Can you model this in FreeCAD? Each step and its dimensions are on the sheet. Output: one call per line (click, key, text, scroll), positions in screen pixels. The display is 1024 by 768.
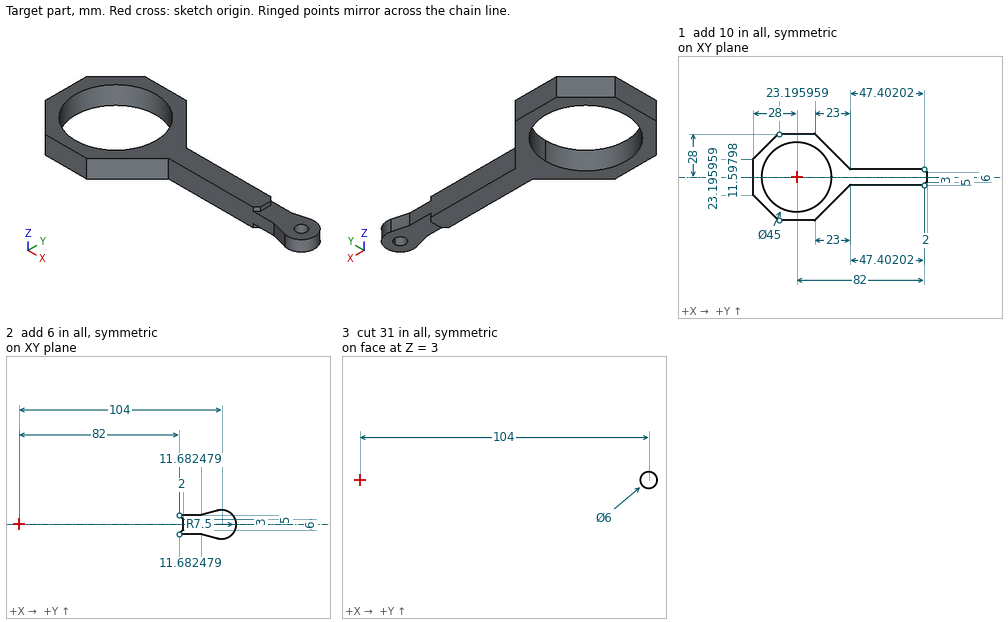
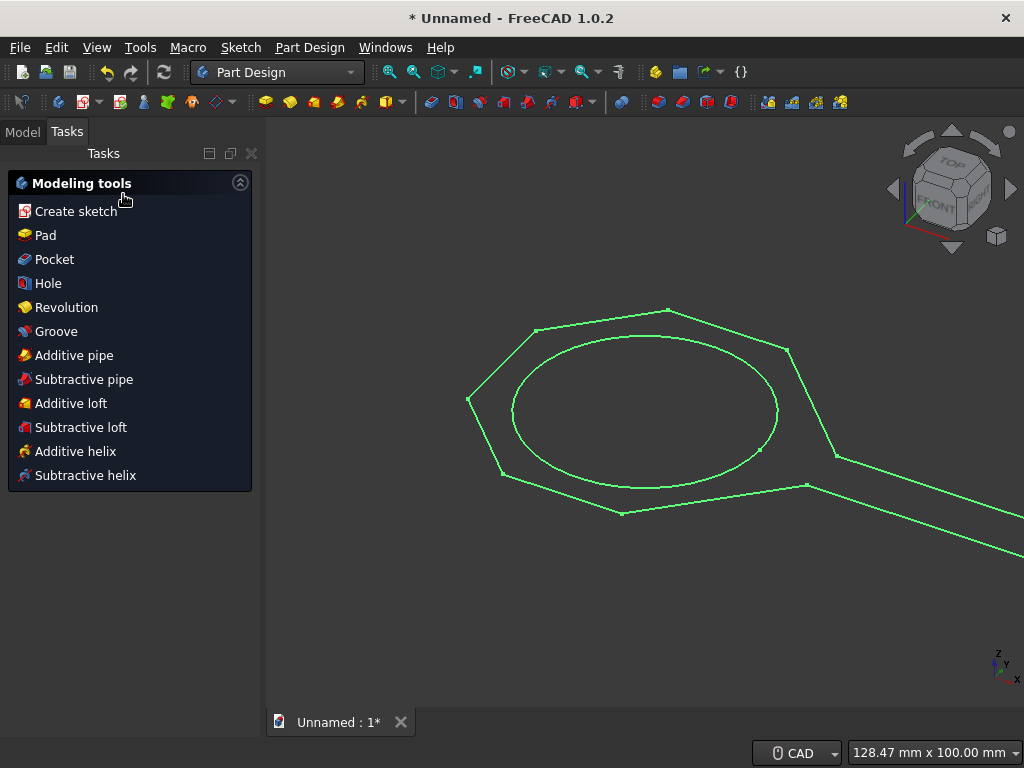
click(266, 102)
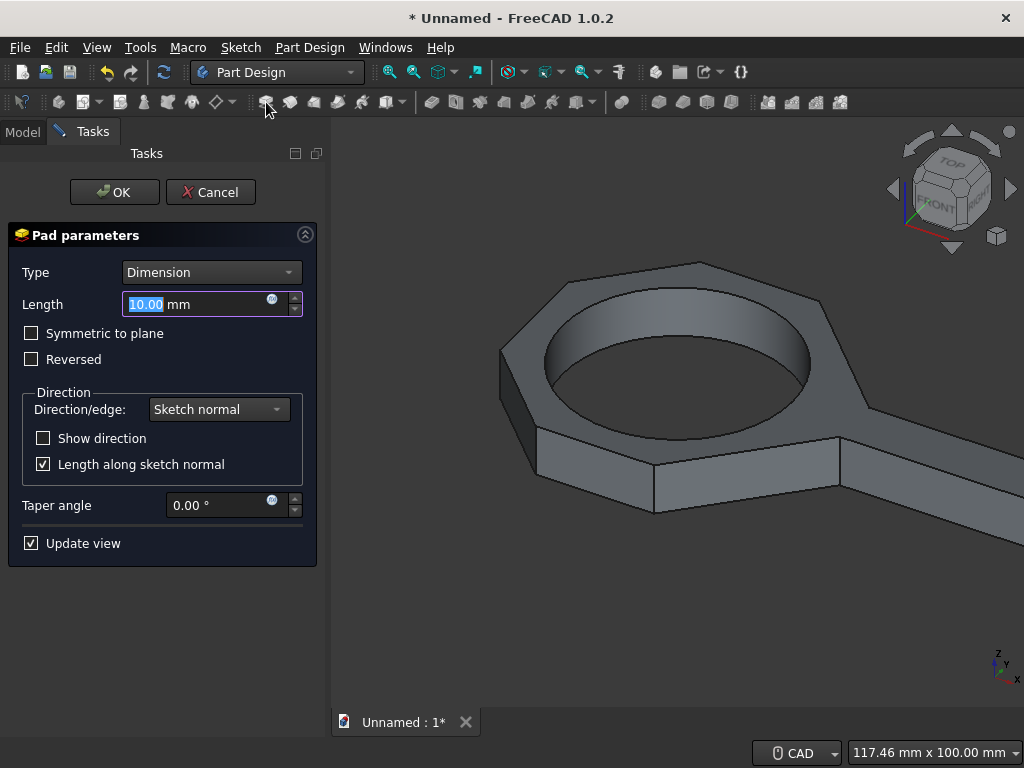
text(10)
key(Tab)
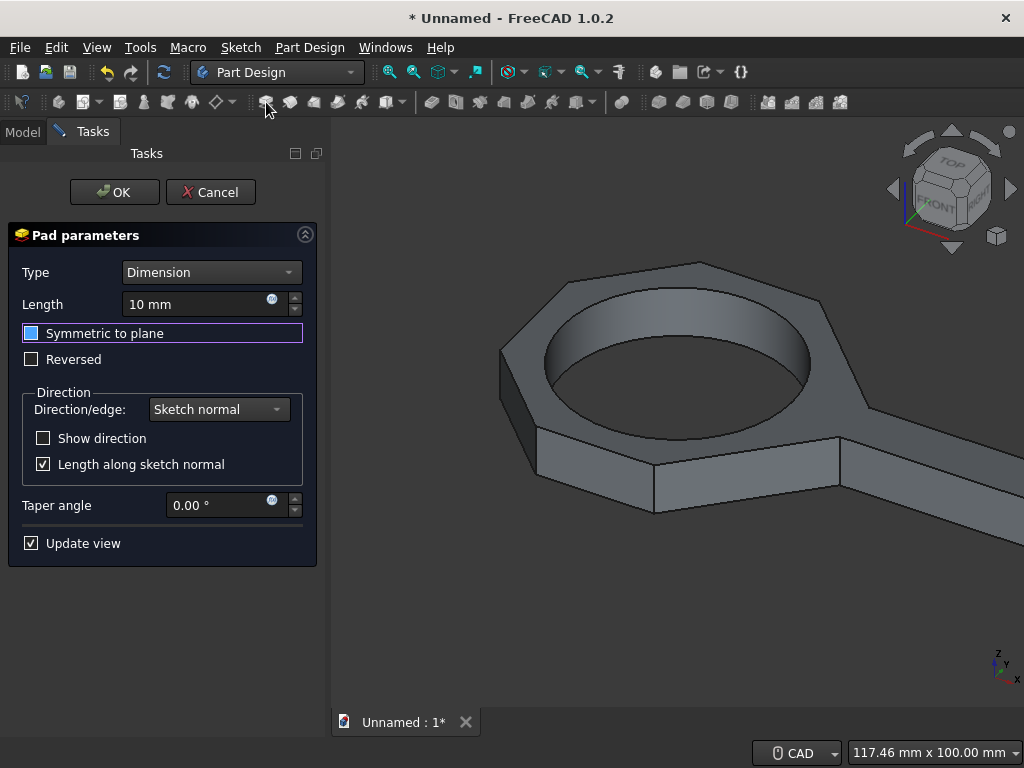
click(30, 333)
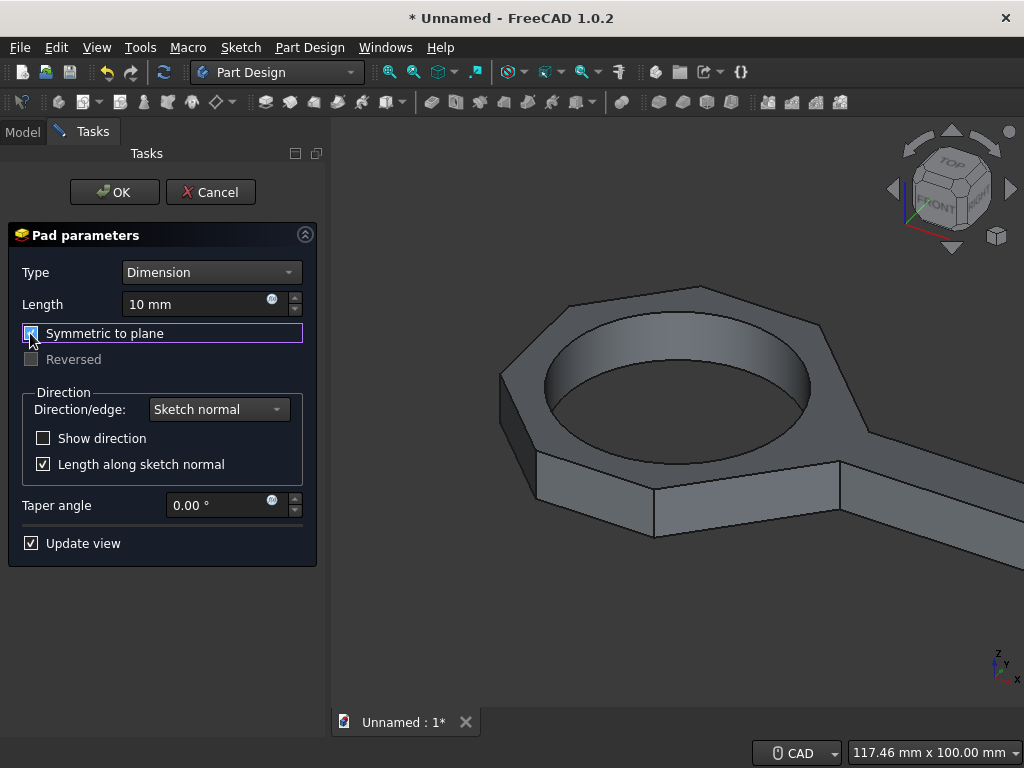
click(115, 192)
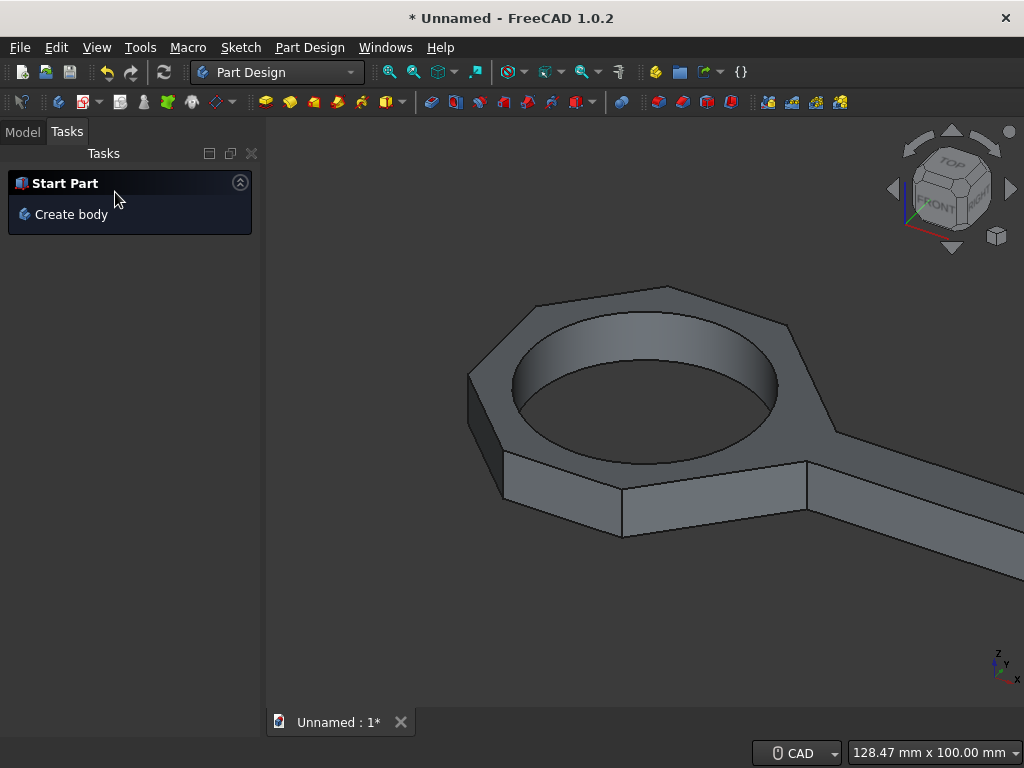
click(390, 72)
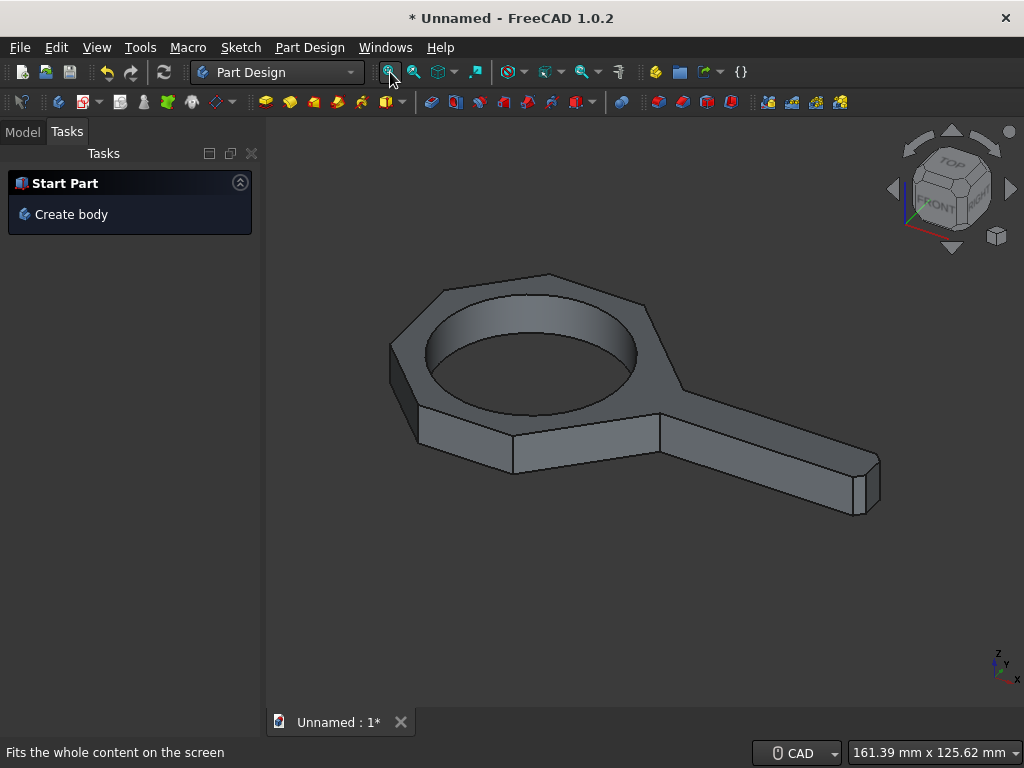
click(84, 102)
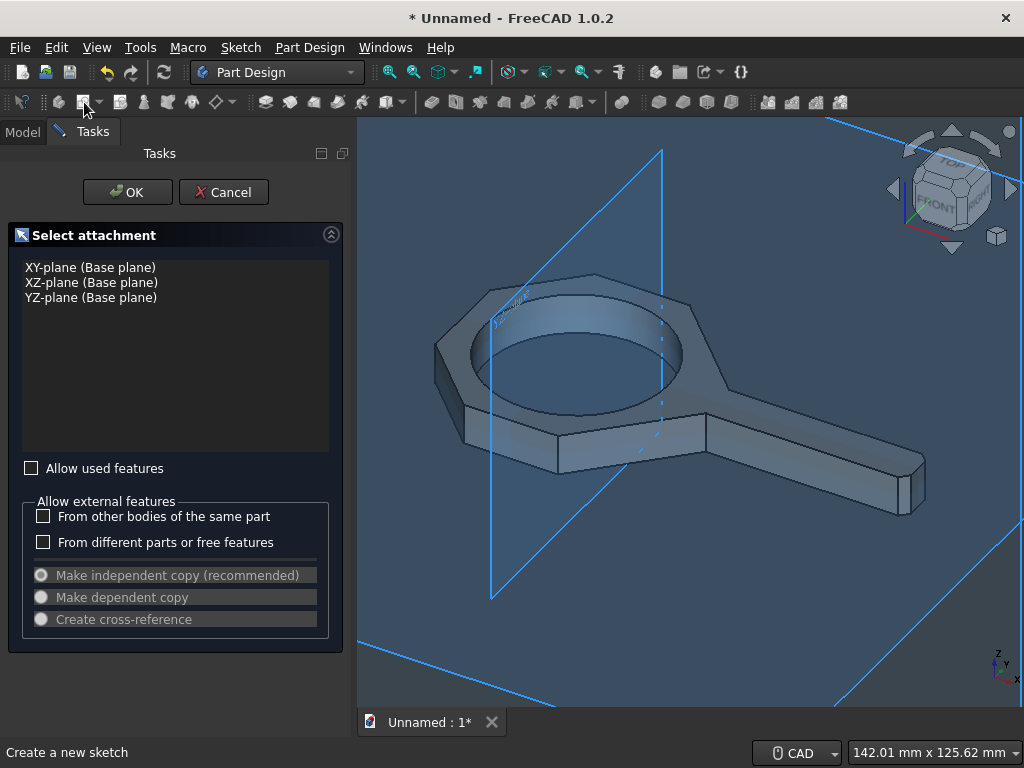
click(82, 268)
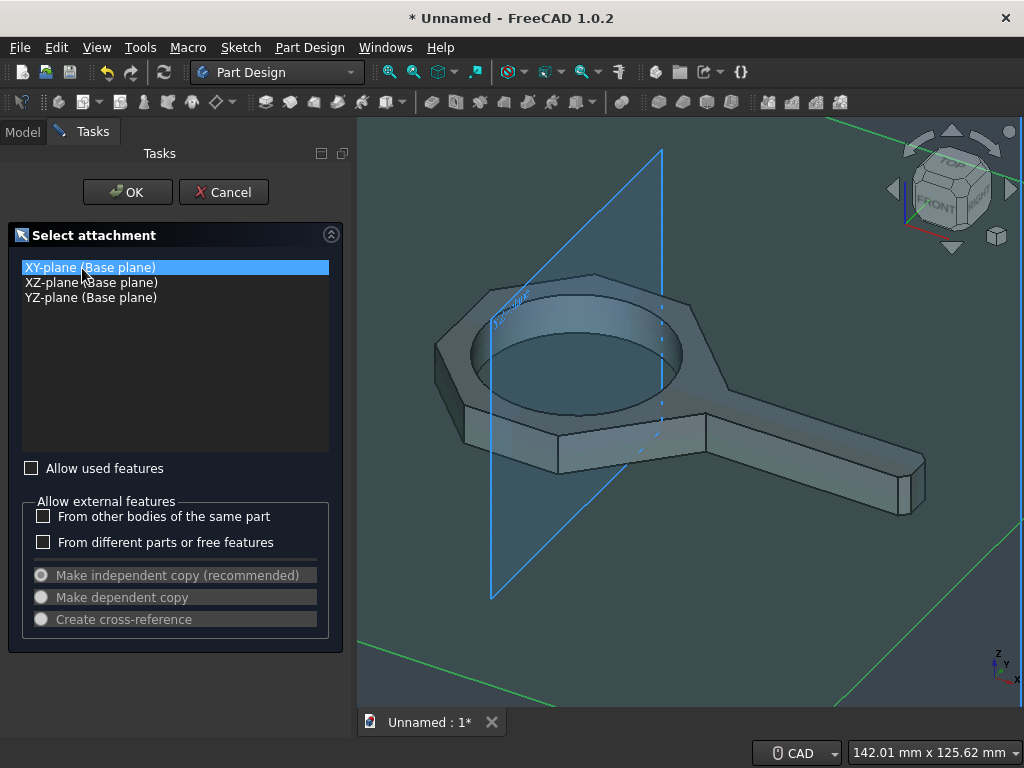
click(128, 192)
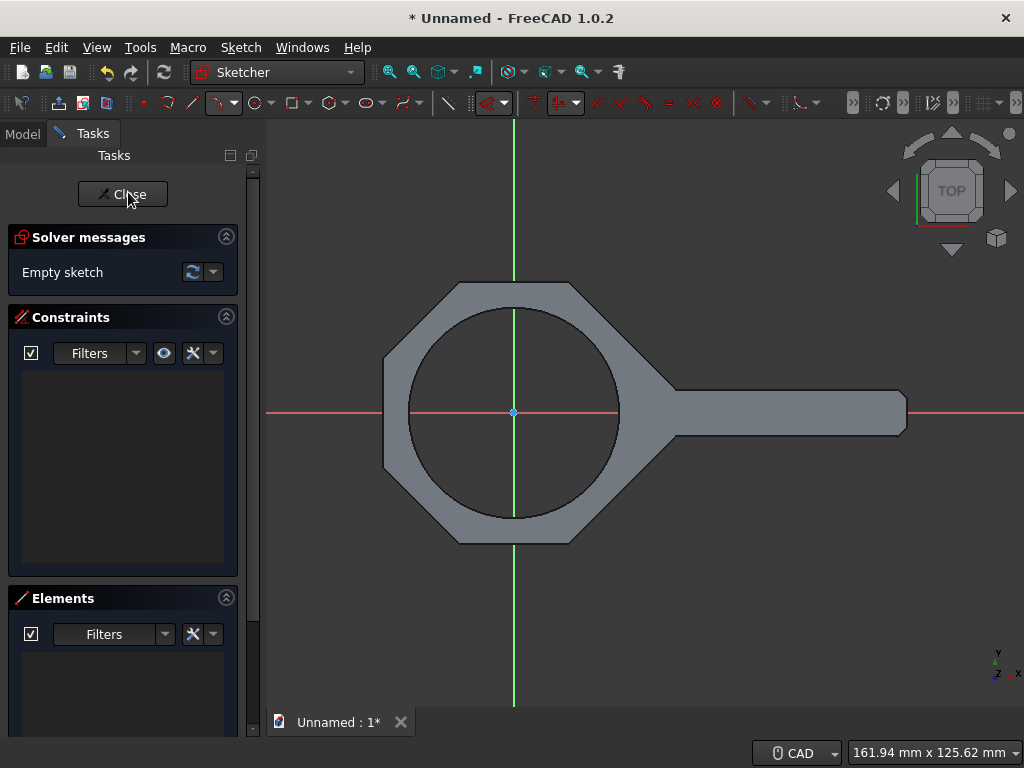
click(108, 104)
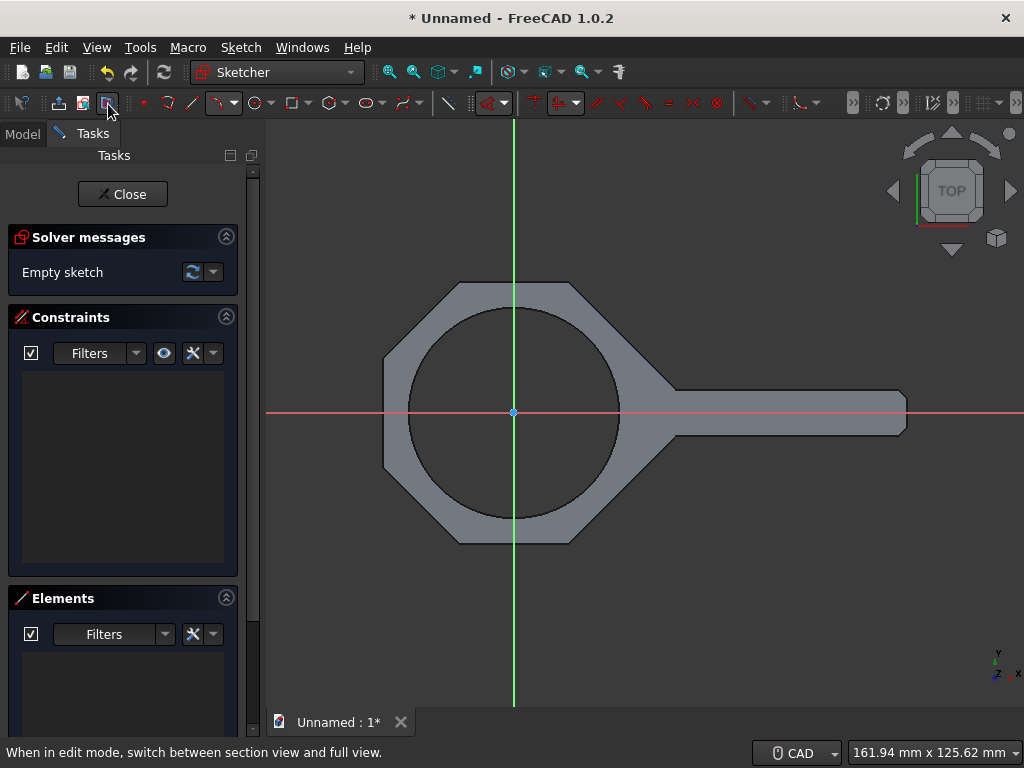
scroll(576, 413, down, 5)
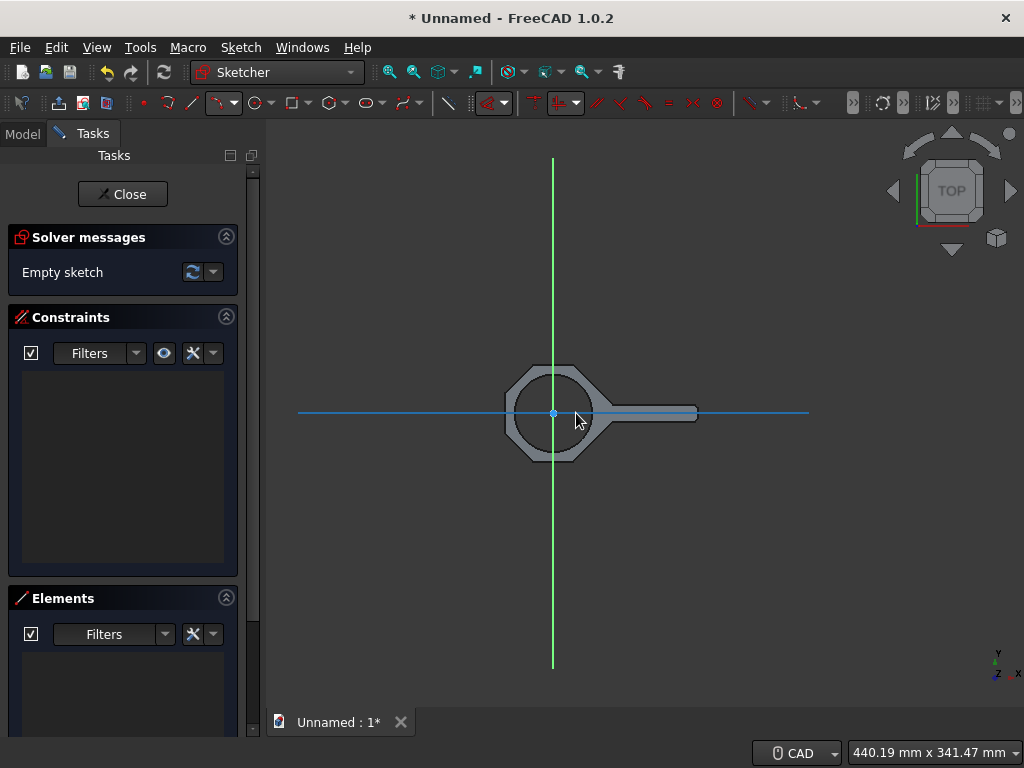
scroll(742, 413, up, 10)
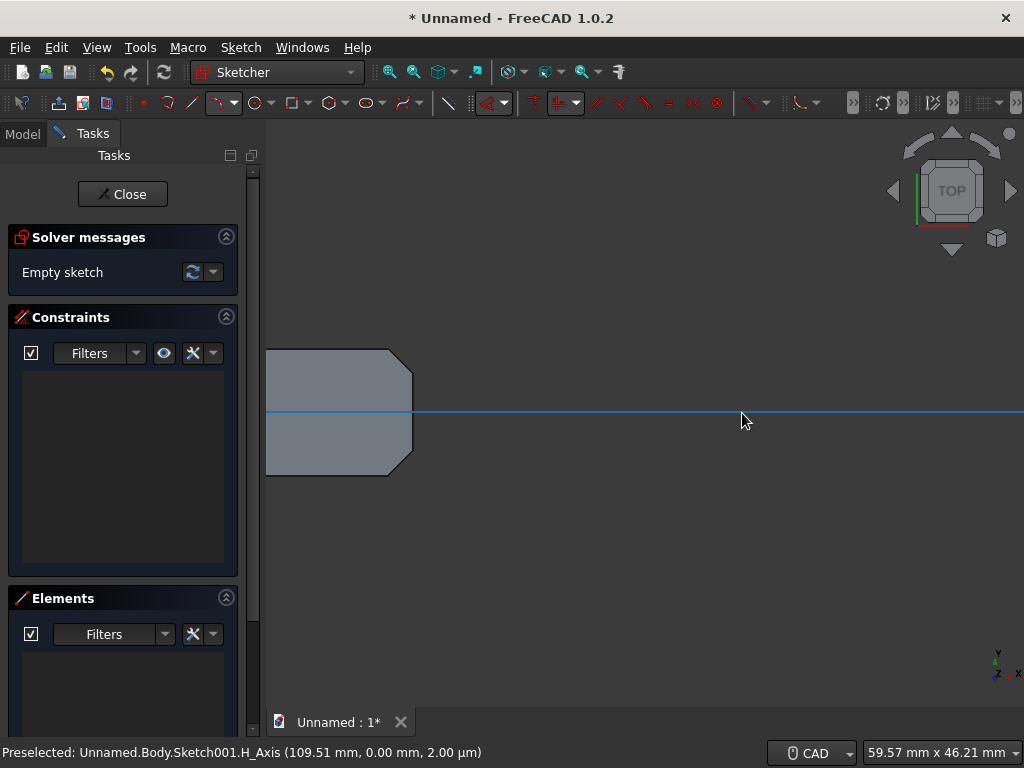
click(168, 104)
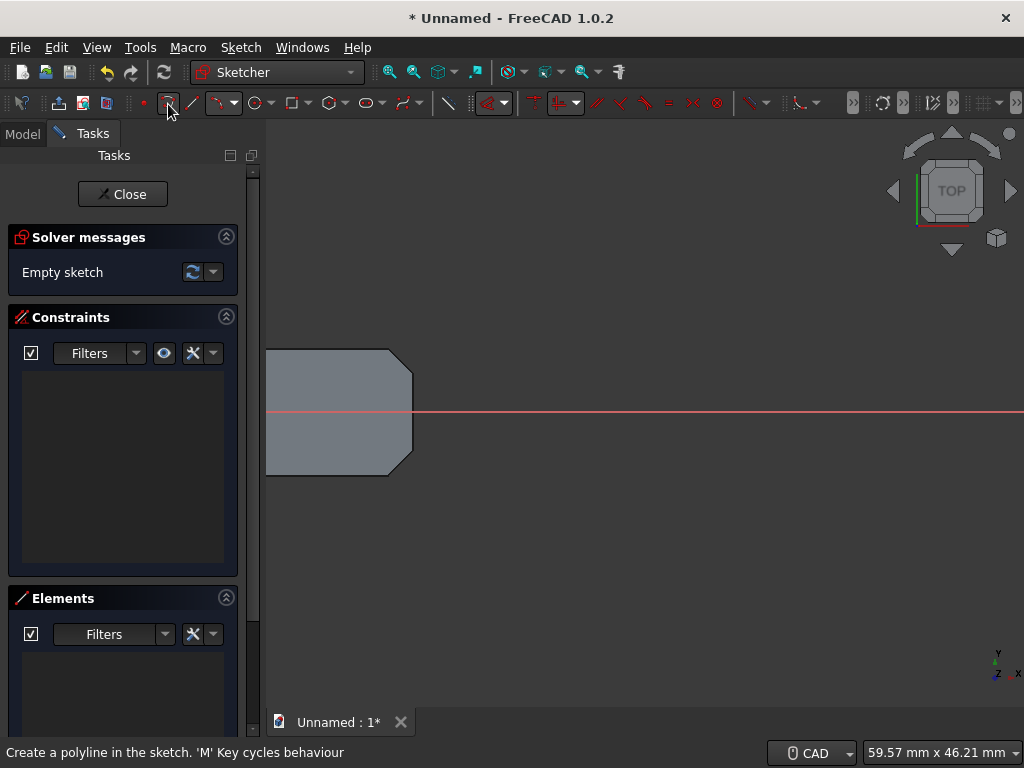
click(643, 320)
click(537, 349)
click(388, 349)
click(413, 374)
click(413, 450)
click(388, 476)
click(537, 476)
click(643, 504)
right_click(643, 504)